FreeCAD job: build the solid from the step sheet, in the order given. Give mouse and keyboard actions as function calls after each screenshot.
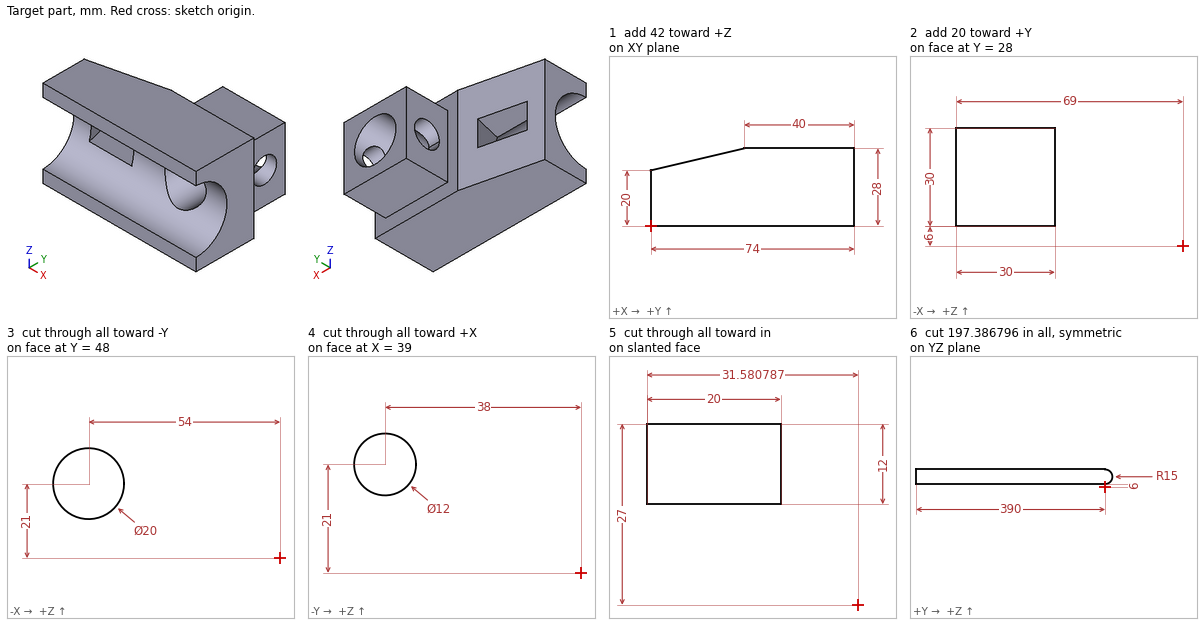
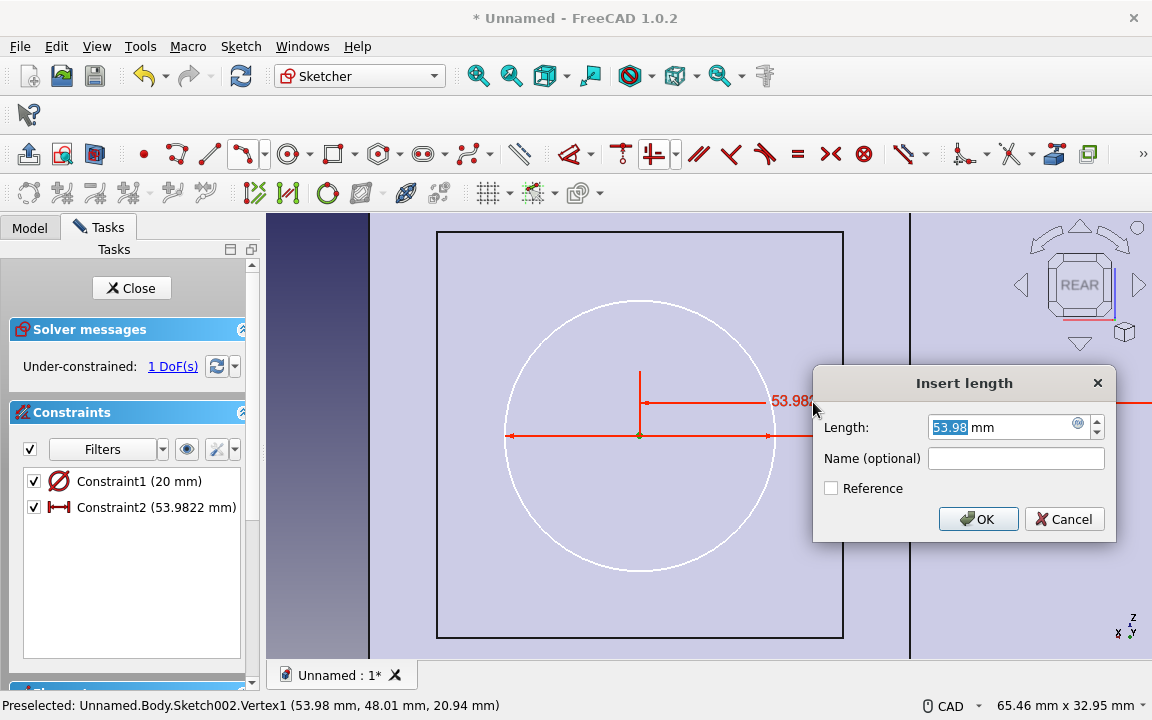
text(54)
key(Return)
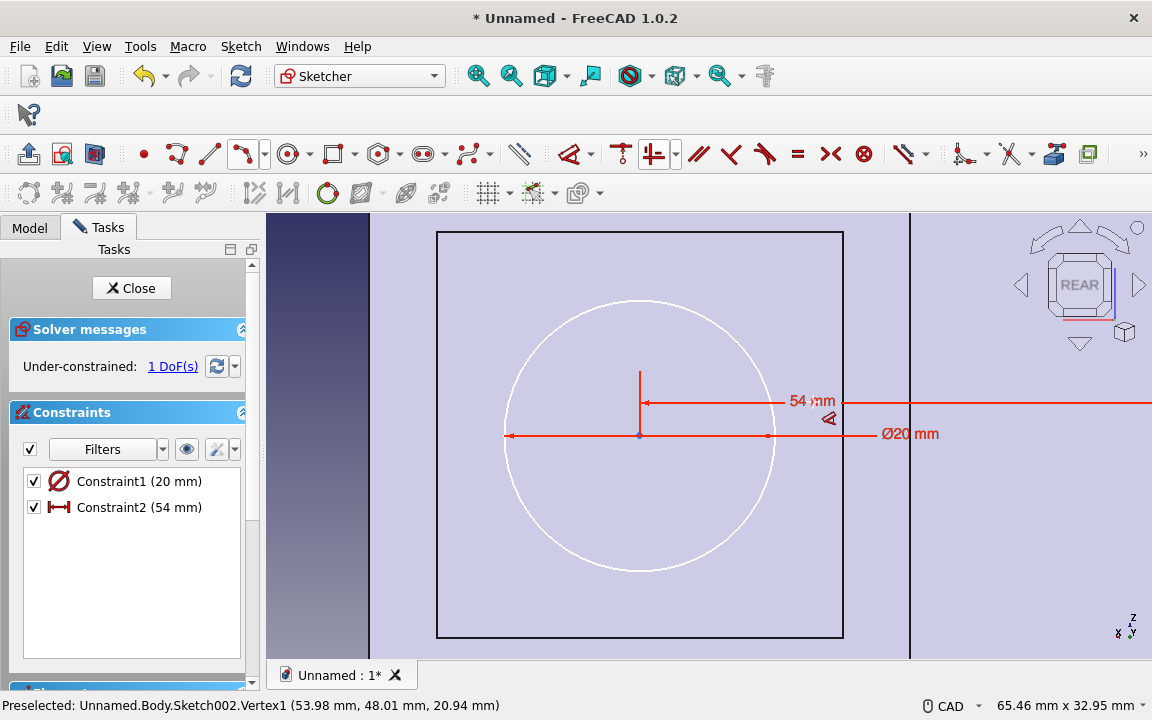
click(640, 436)
click(606, 534)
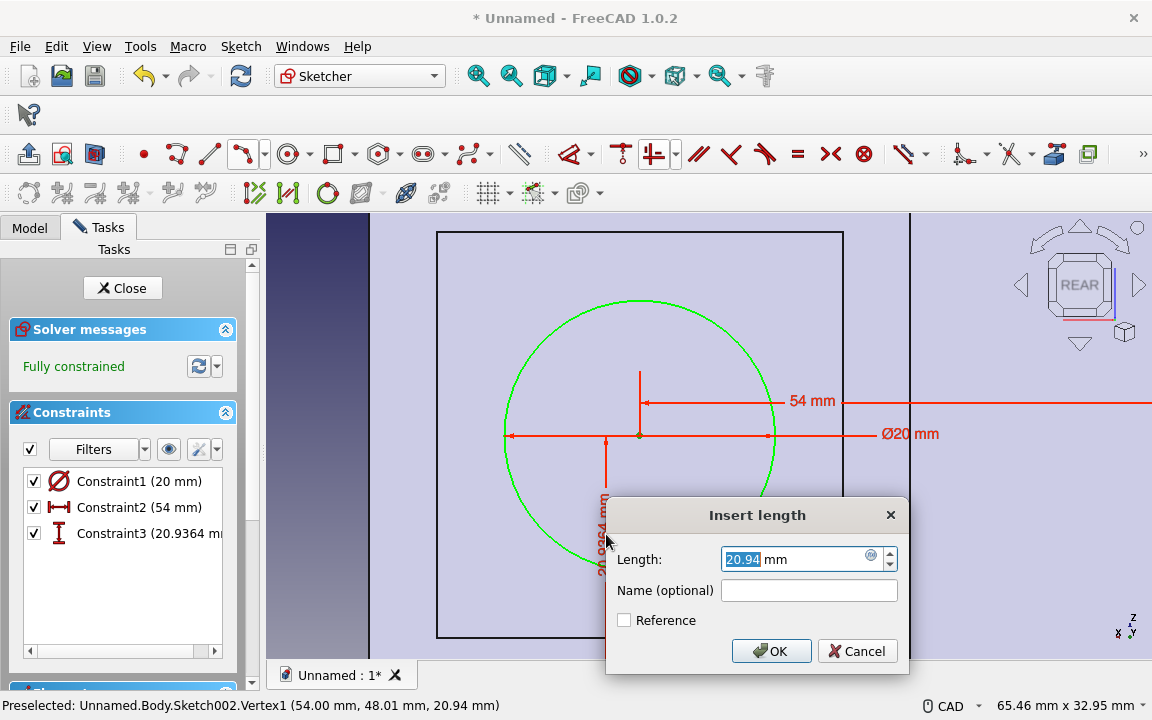
text(21)
key(Return)
key(Escape)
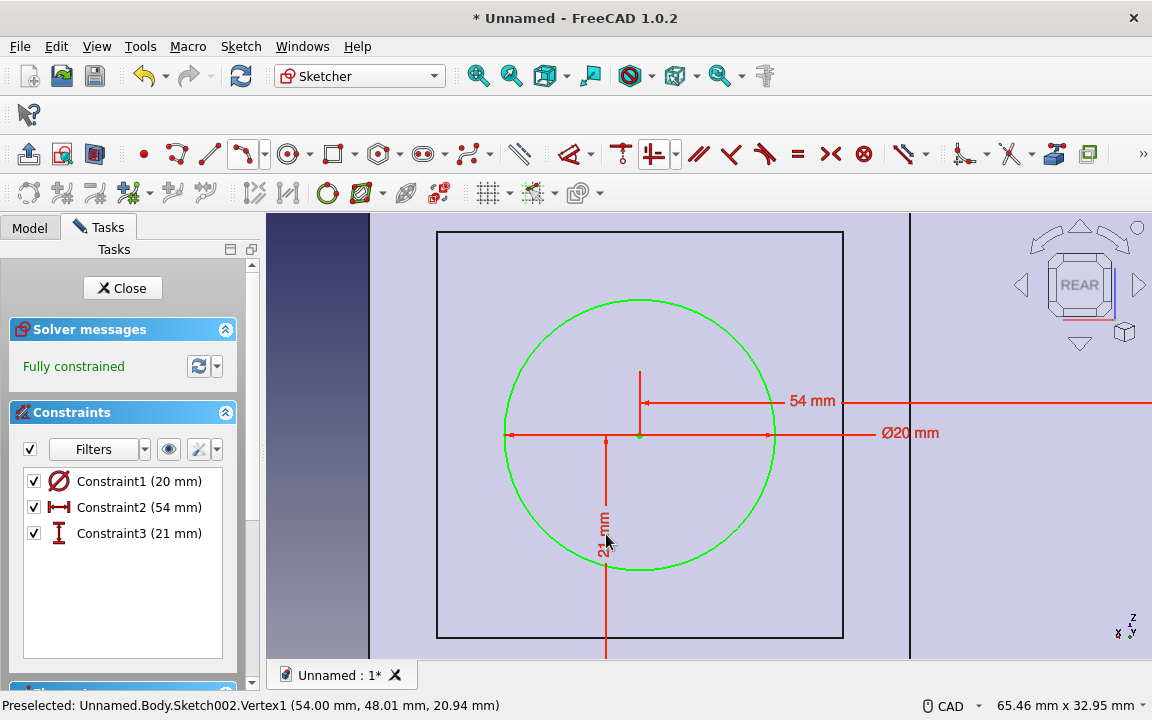
click(123, 288)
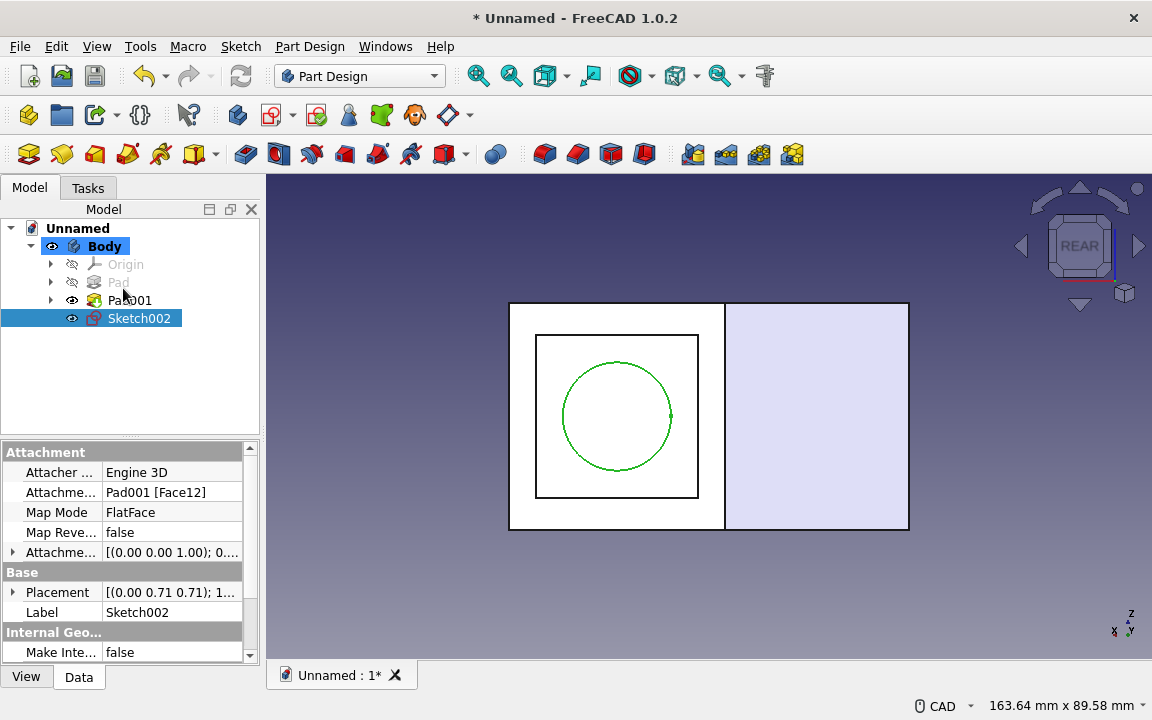
click(246, 154)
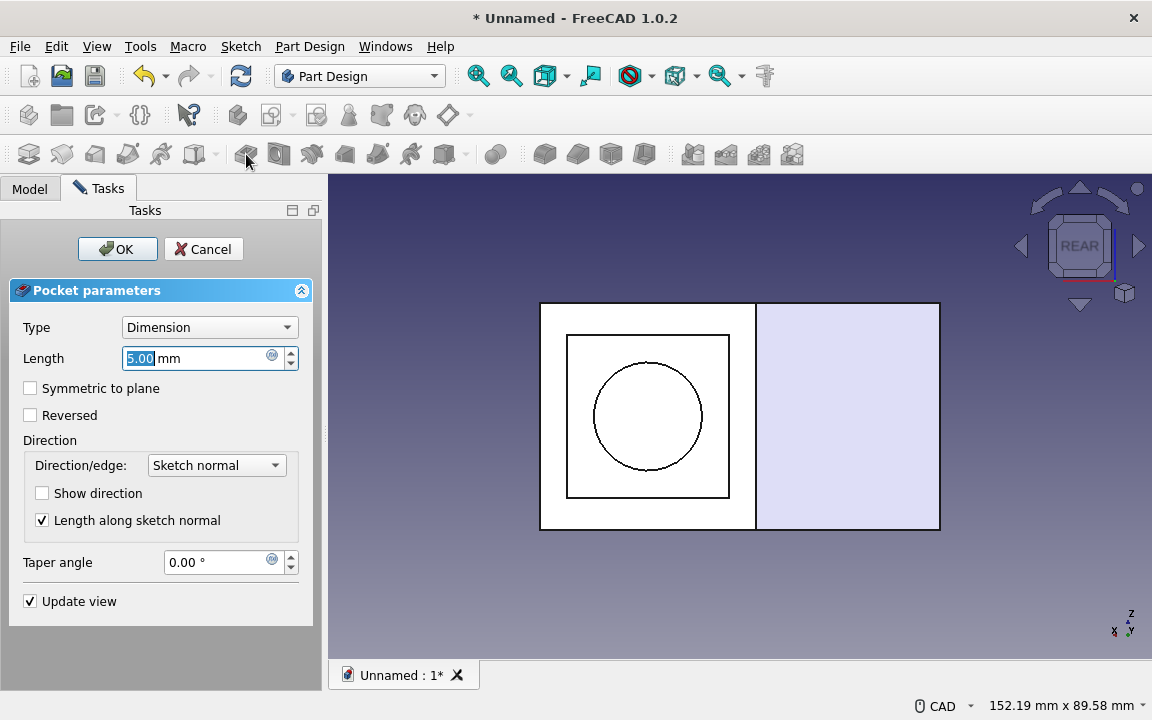
click(210, 328)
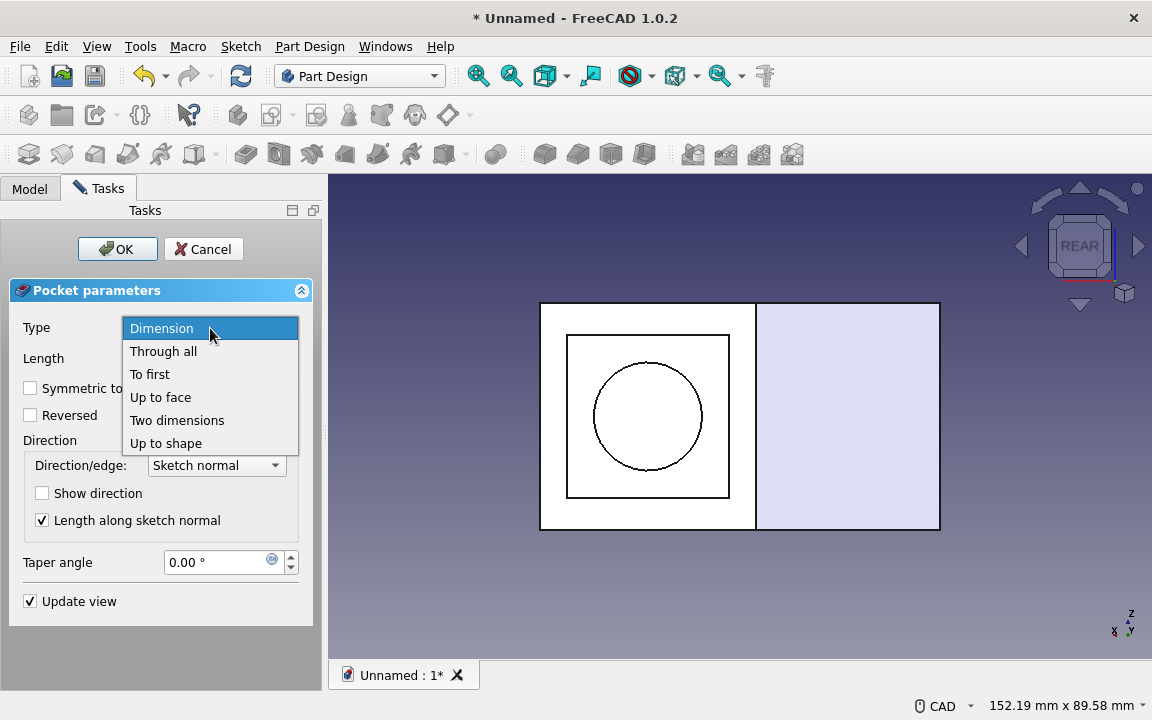
click(208, 352)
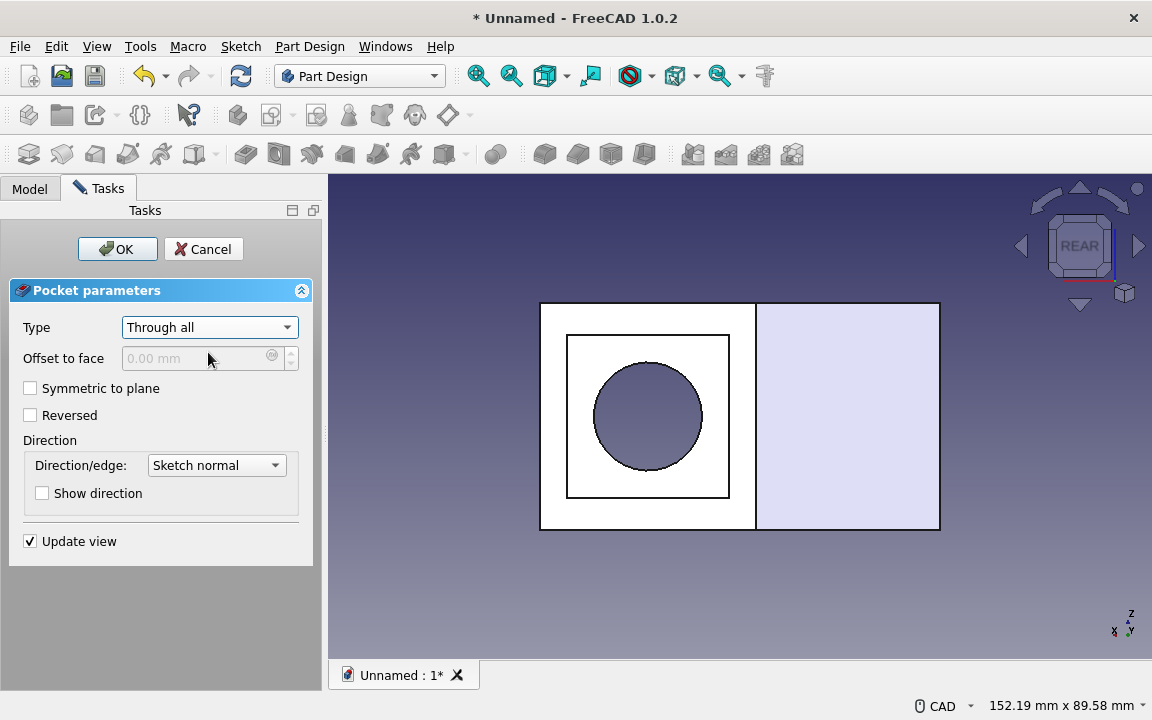
click(118, 249)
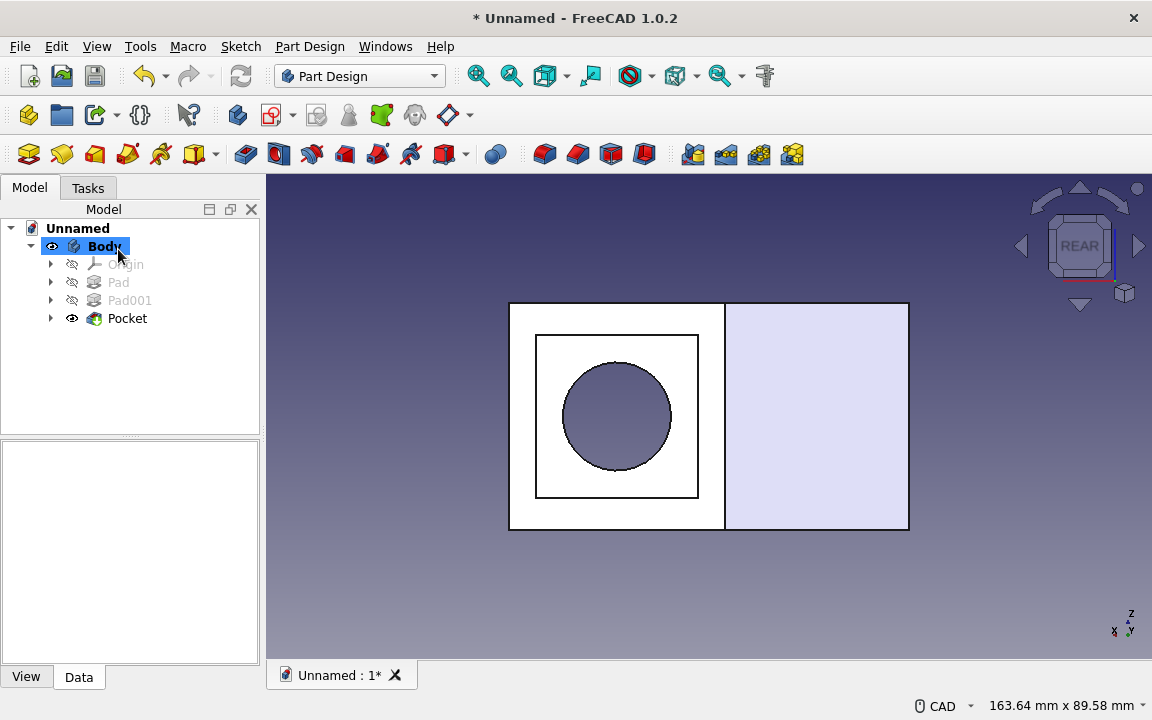
key(6)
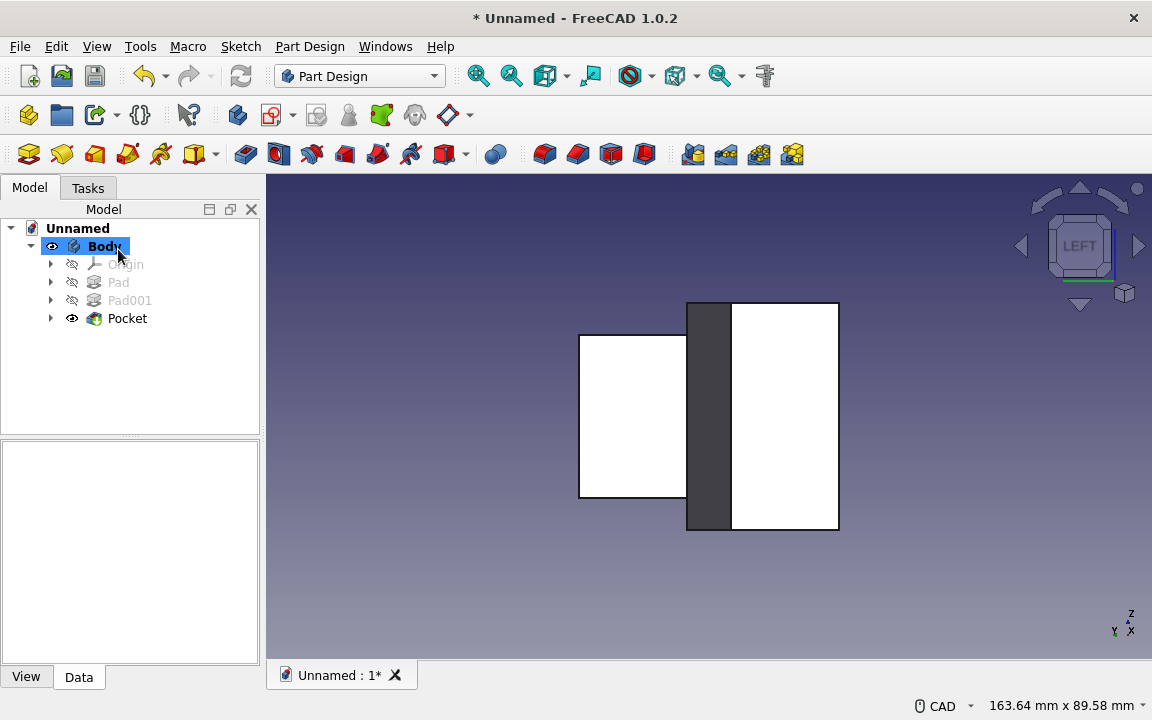
click(633, 392)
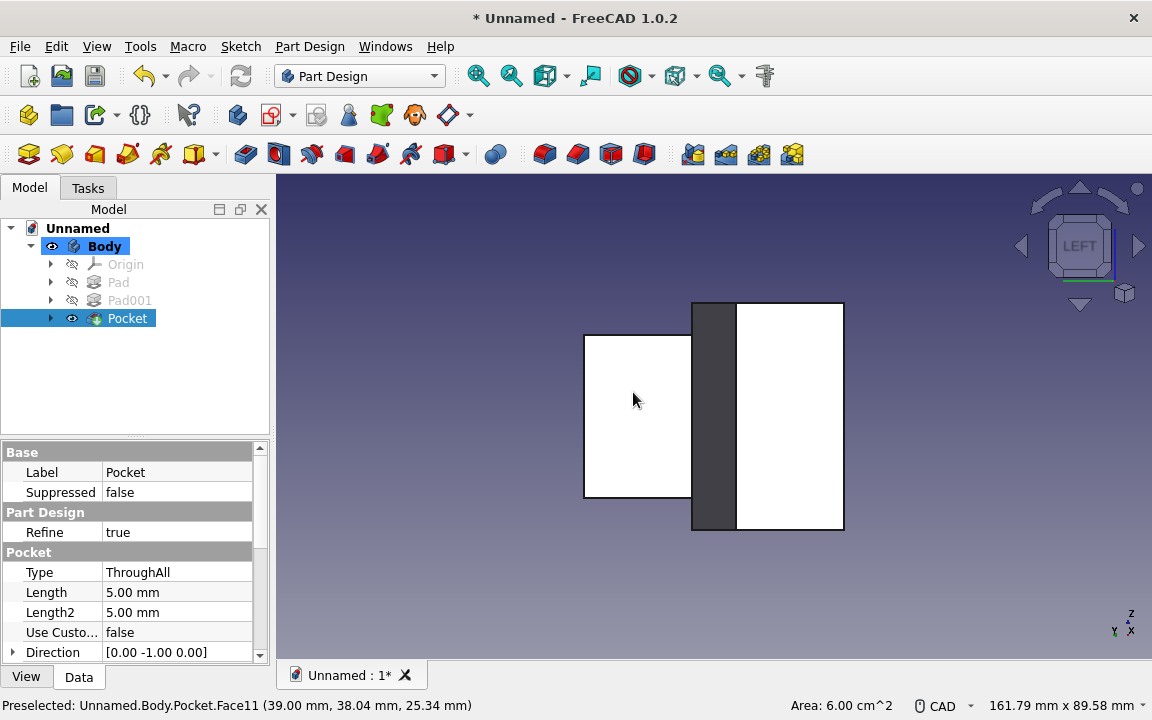
click(270, 116)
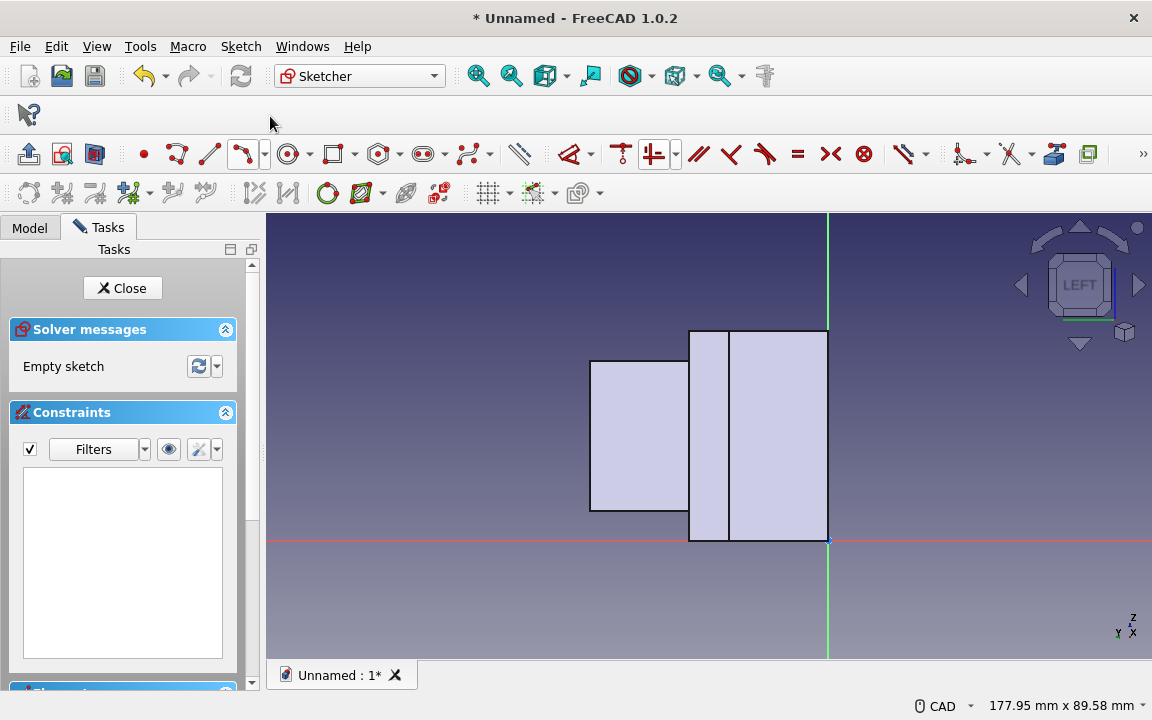
scroll(639, 436, up, 8)